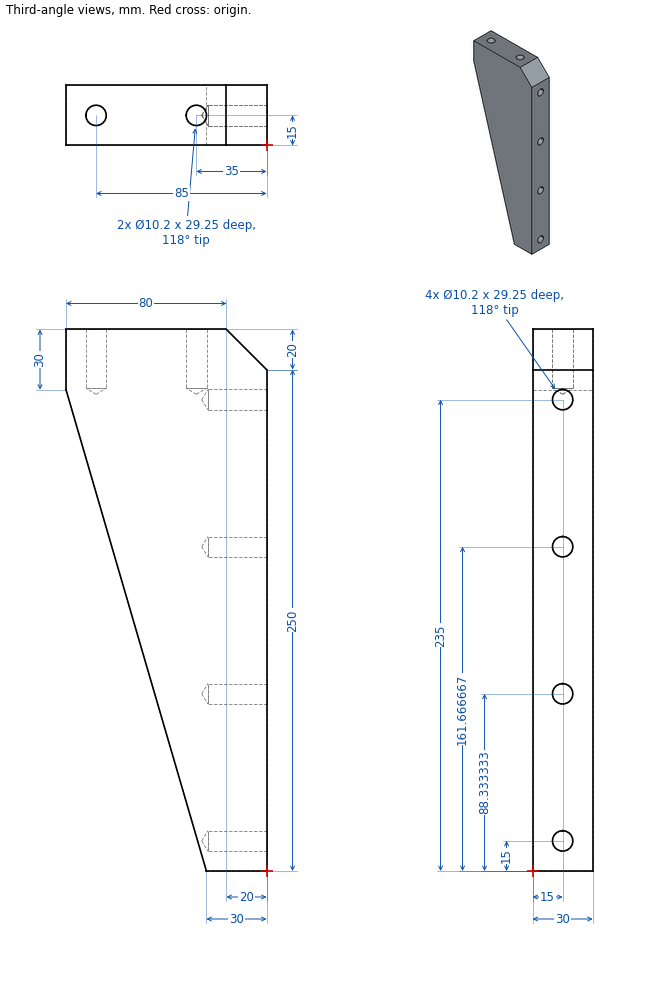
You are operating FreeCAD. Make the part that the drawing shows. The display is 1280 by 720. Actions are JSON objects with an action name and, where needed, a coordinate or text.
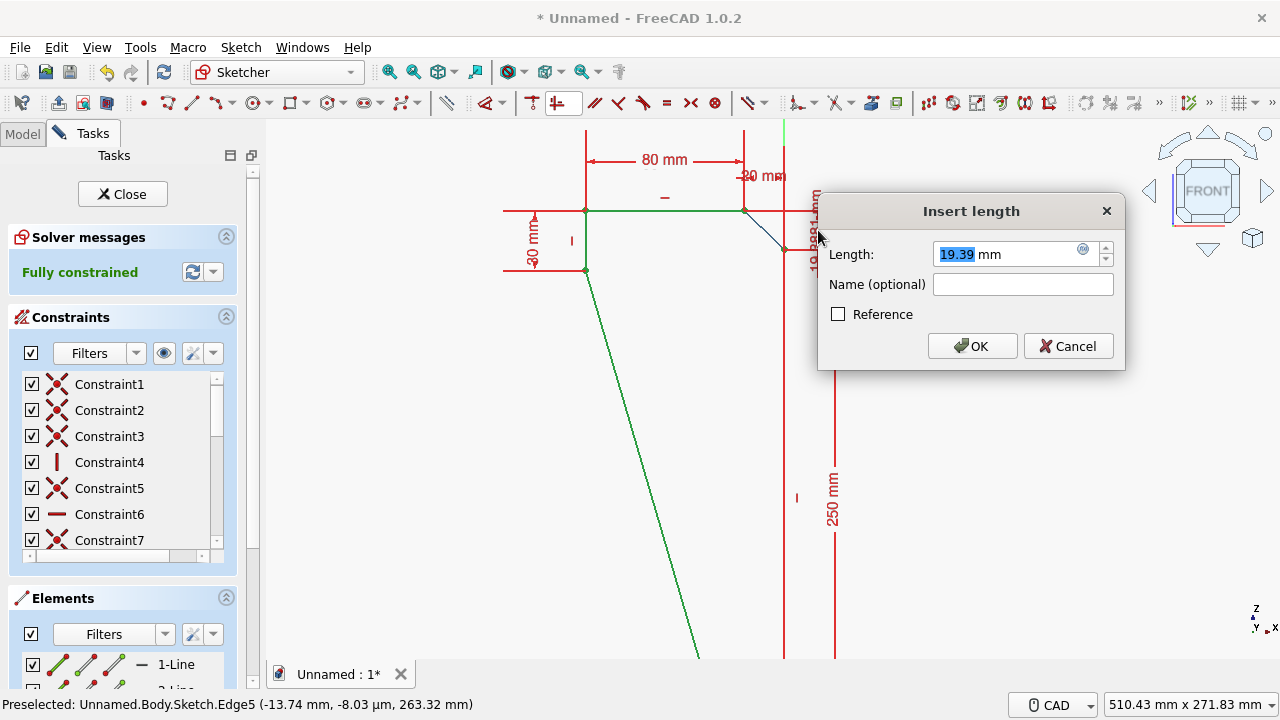
{"action": "type", "text": "20"}
{"action": "key", "text": "Return"}
{"action": "key", "text": "Escape"}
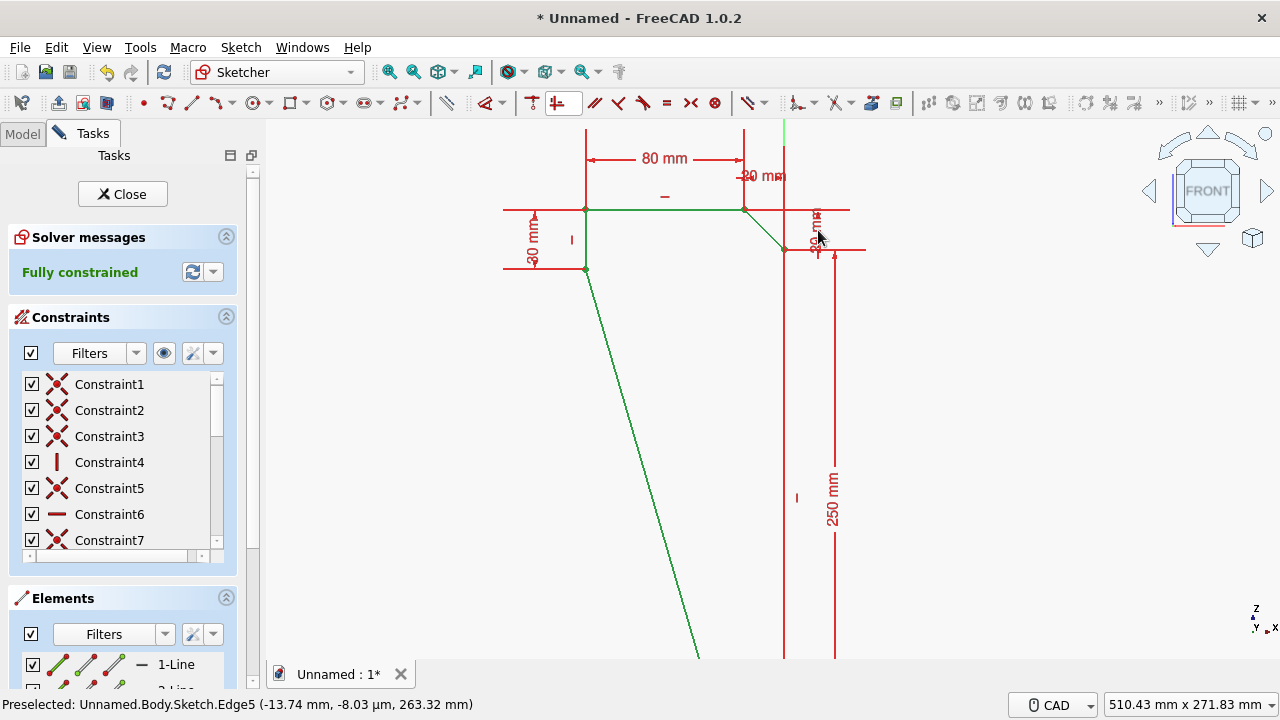
{"action": "left_click", "coordinate": [123, 194]}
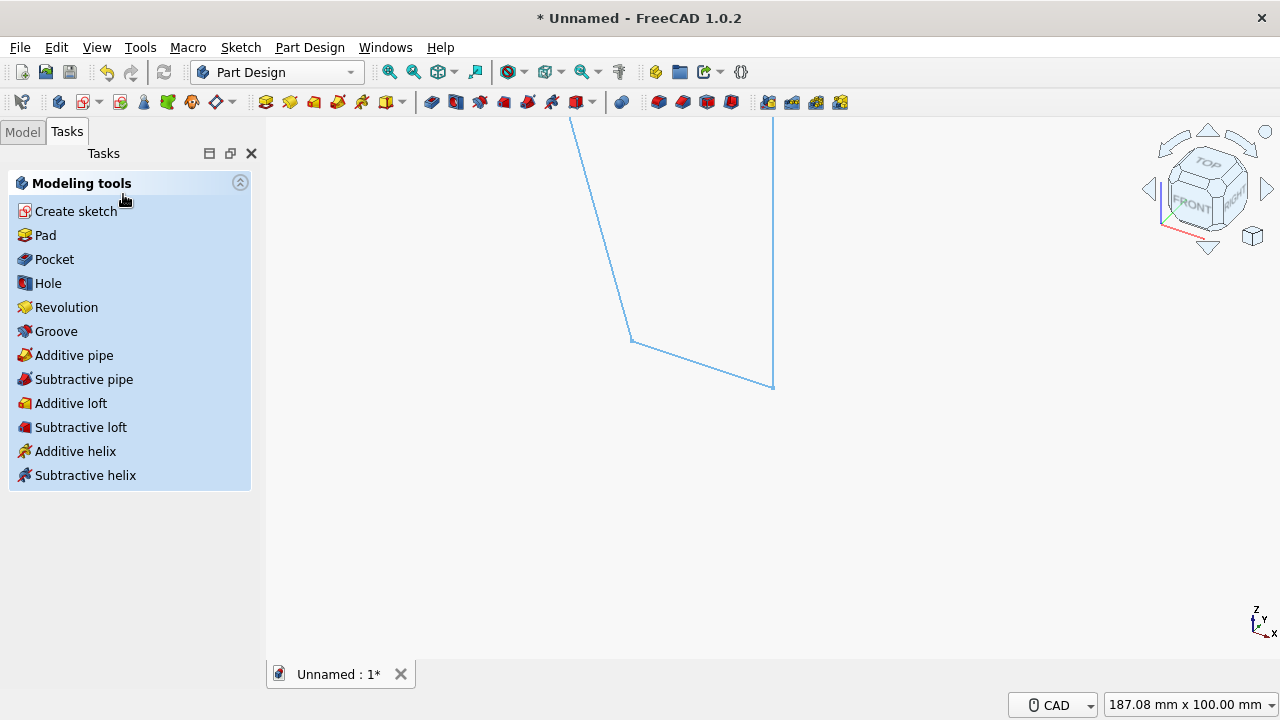
{"action": "left_click", "coordinate": [266, 102]}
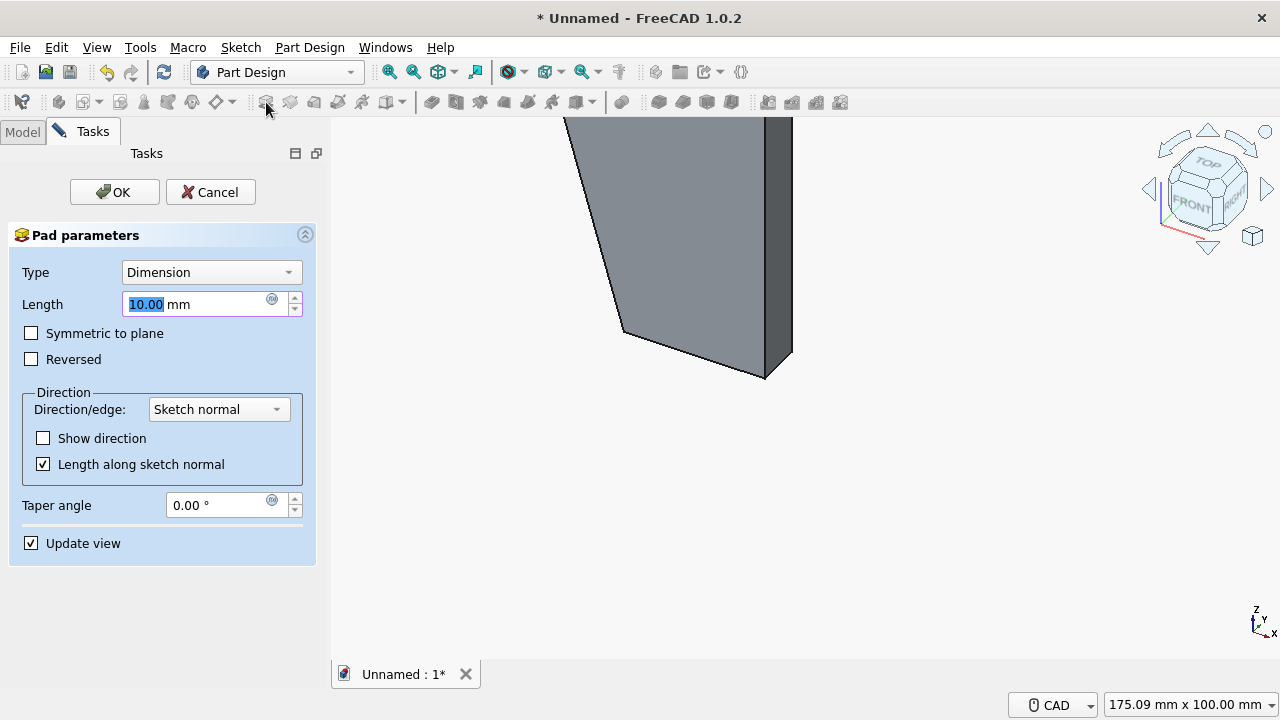
{"action": "type", "text": "30"}
{"action": "key", "text": "Tab"}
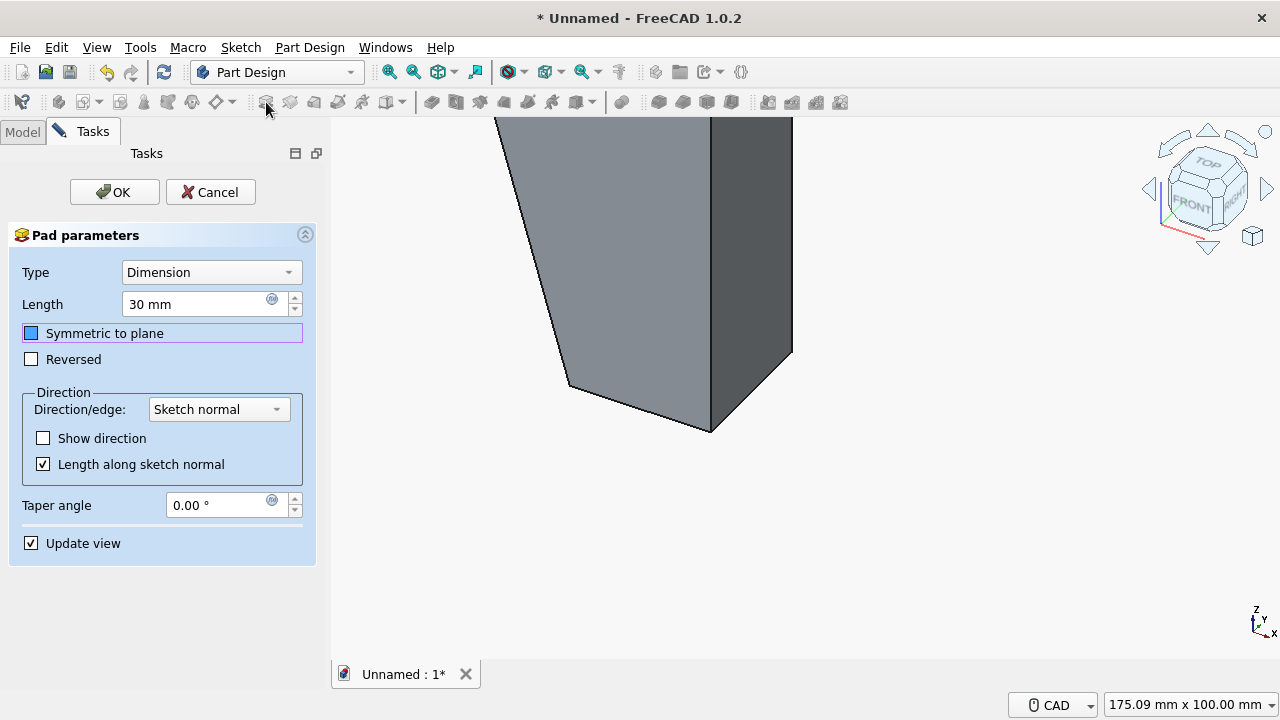
{"action": "left_click", "coordinate": [30, 359]}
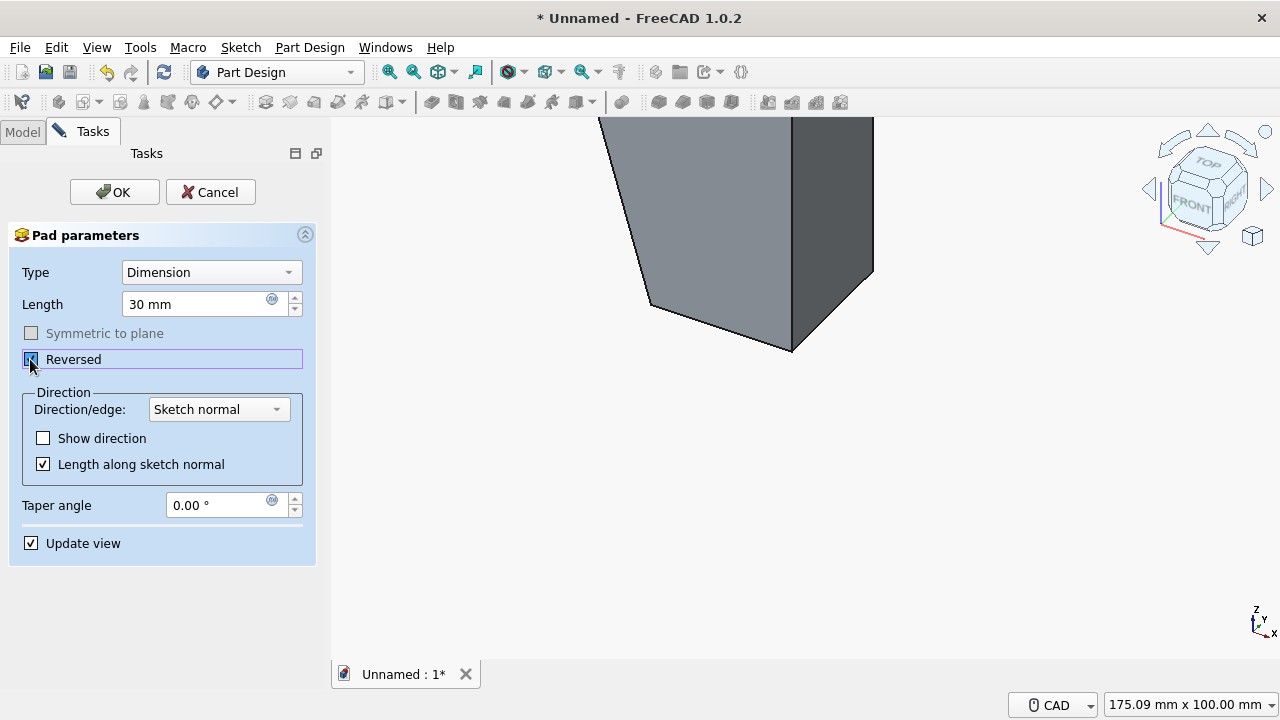
{"action": "left_click", "coordinate": [115, 192]}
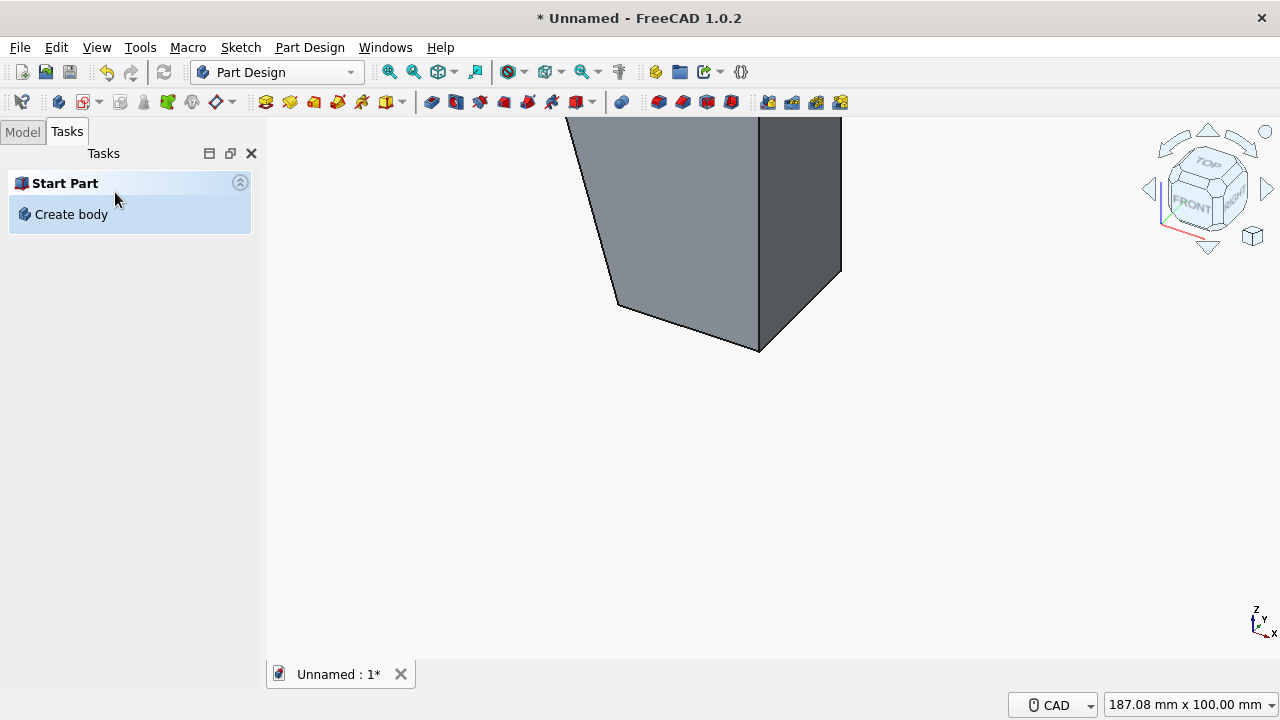
{"action": "left_click", "coordinate": [390, 72]}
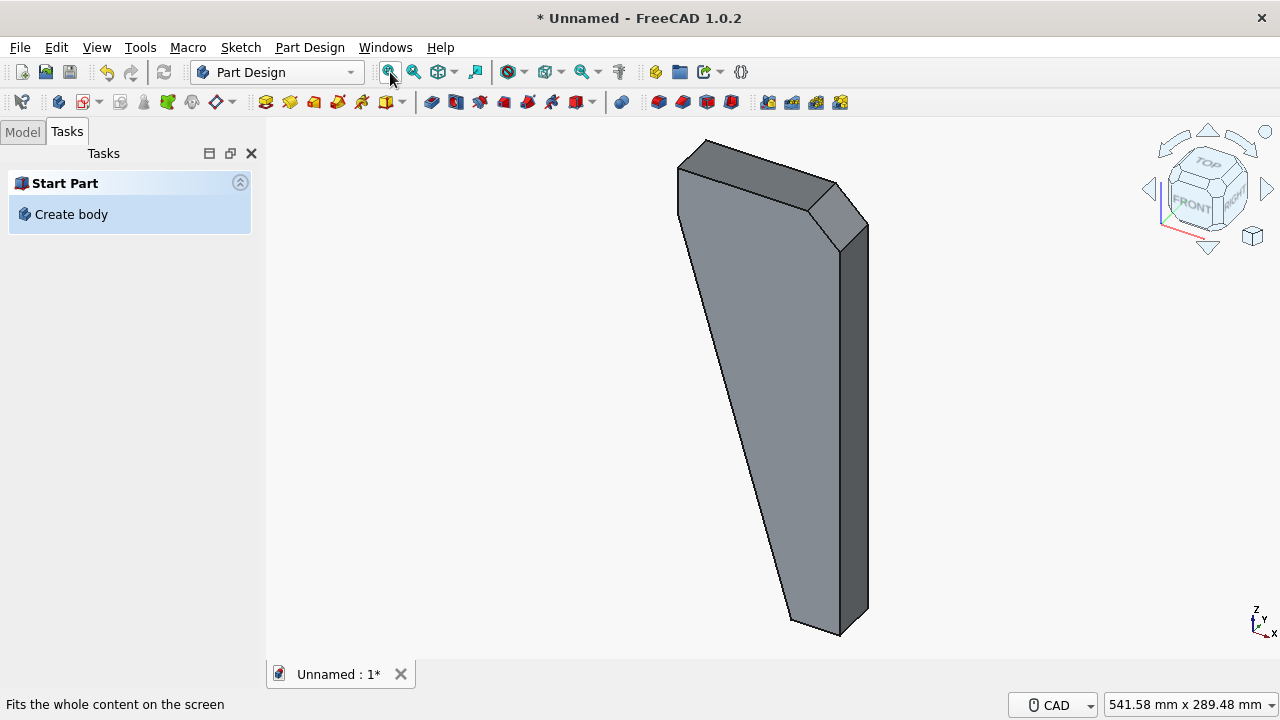
{"action": "left_click", "coordinate": [84, 102]}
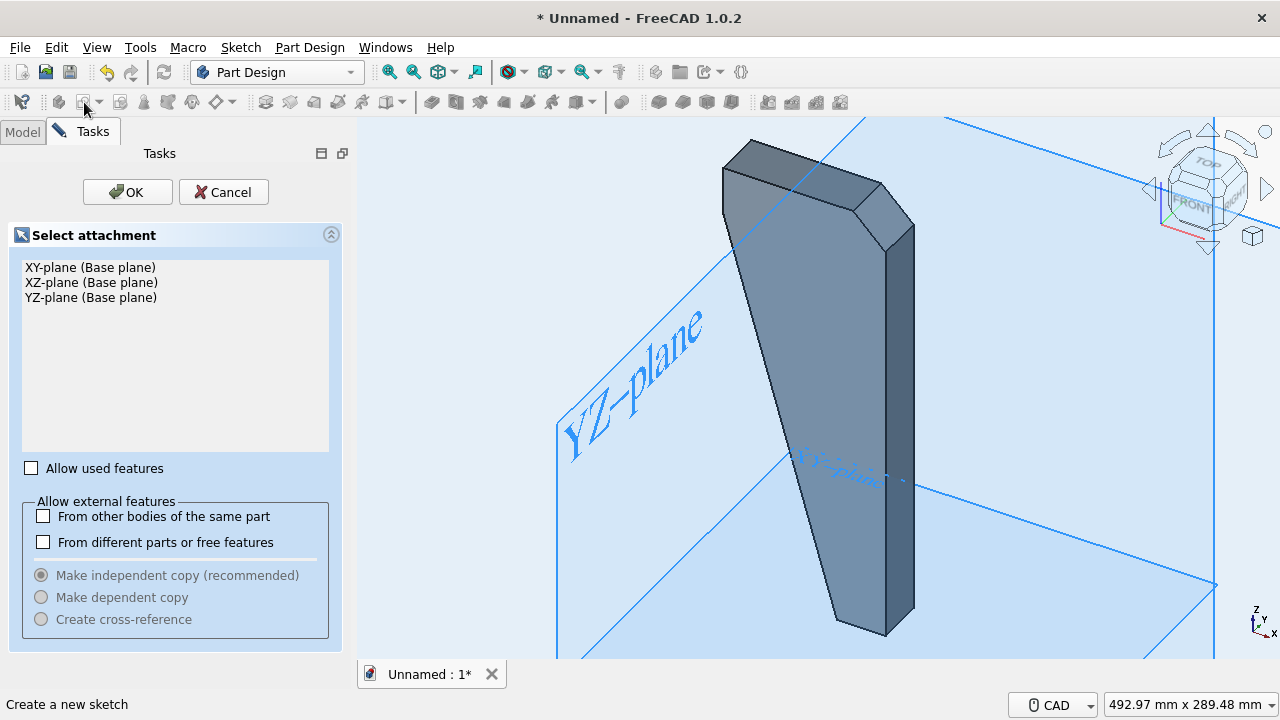
{"action": "left_click", "coordinate": [82, 298]}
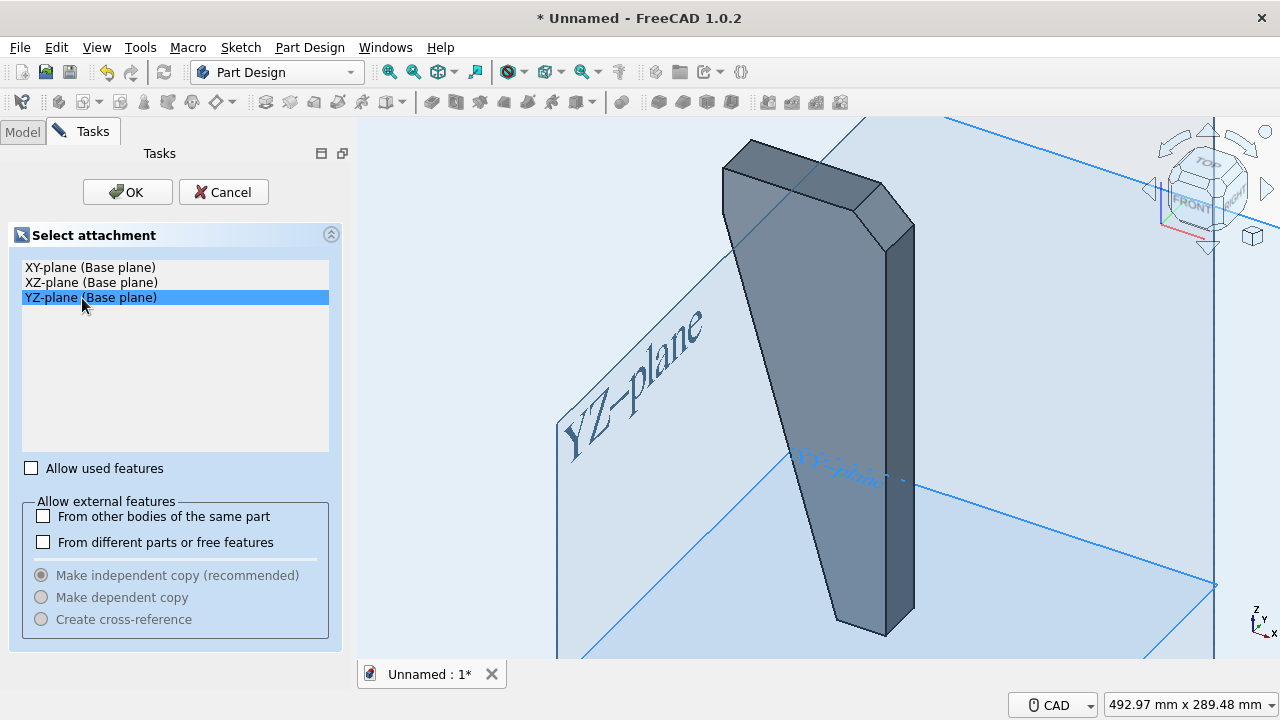
{"action": "left_click", "coordinate": [128, 192]}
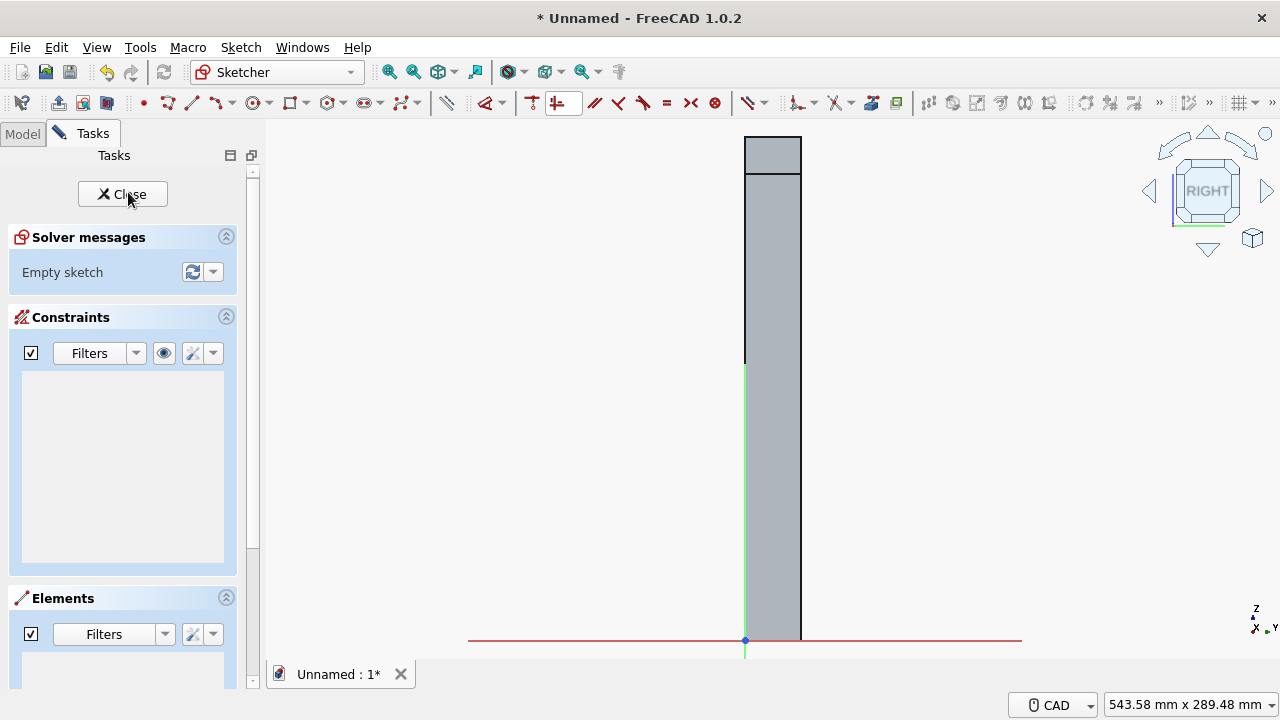
{"action": "scroll", "coordinate": [437, 263], "scroll_direction": "down", "scroll_amount": 1}